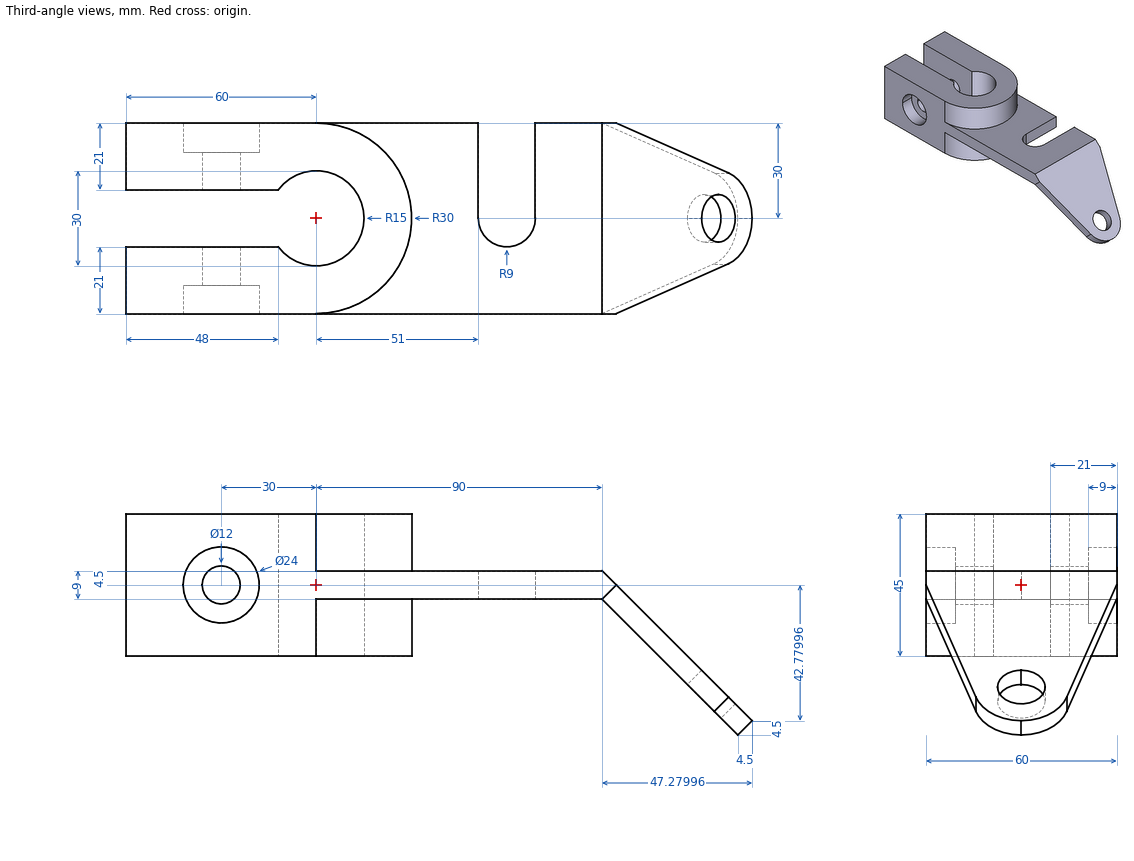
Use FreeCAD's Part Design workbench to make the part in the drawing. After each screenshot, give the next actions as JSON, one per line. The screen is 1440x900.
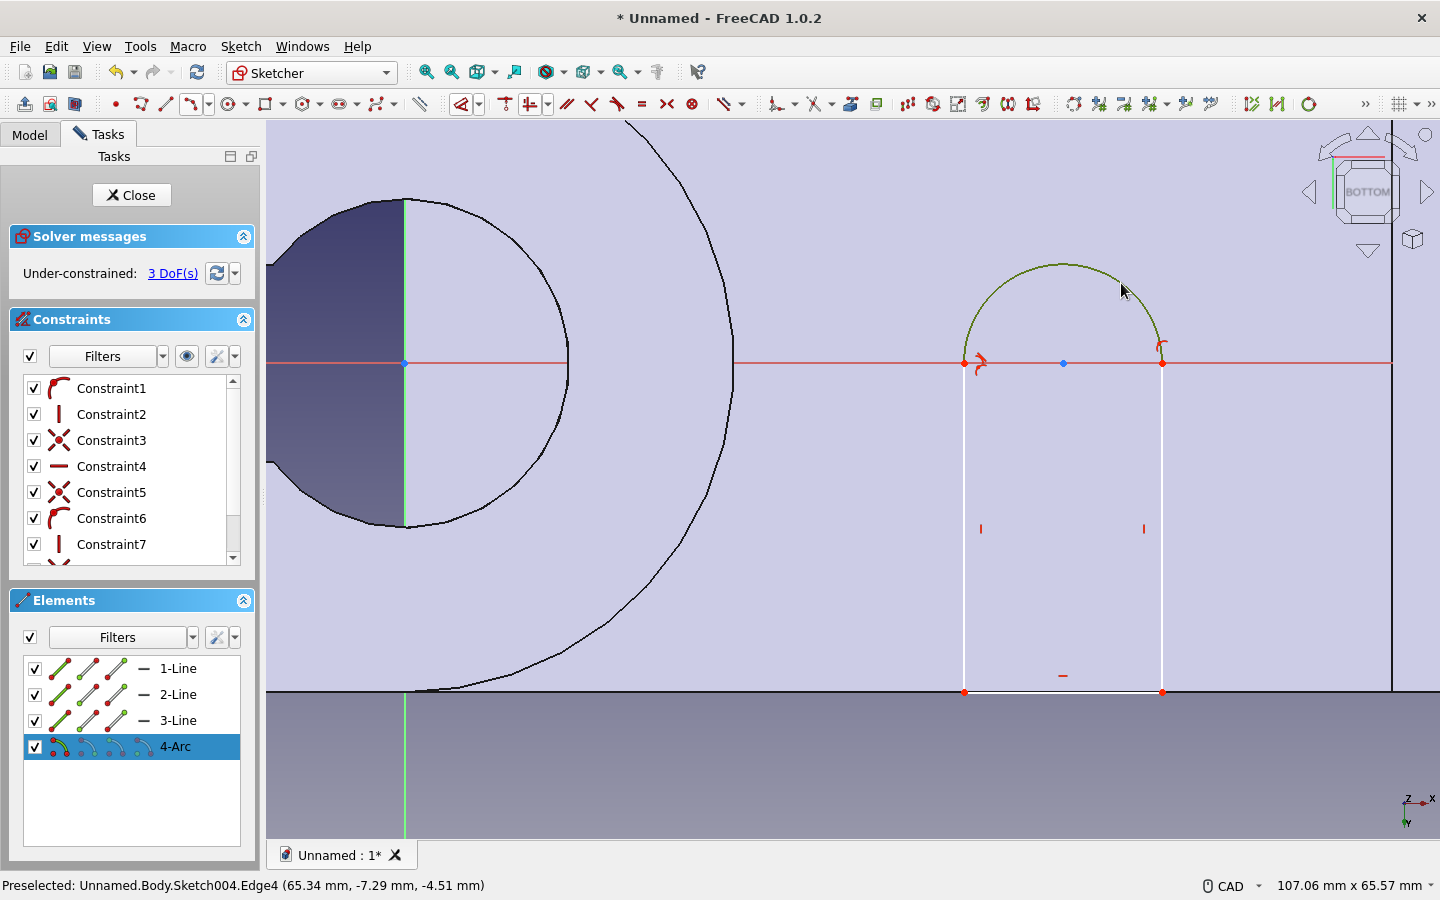
{"action": "left_click", "coordinate": [478, 104]}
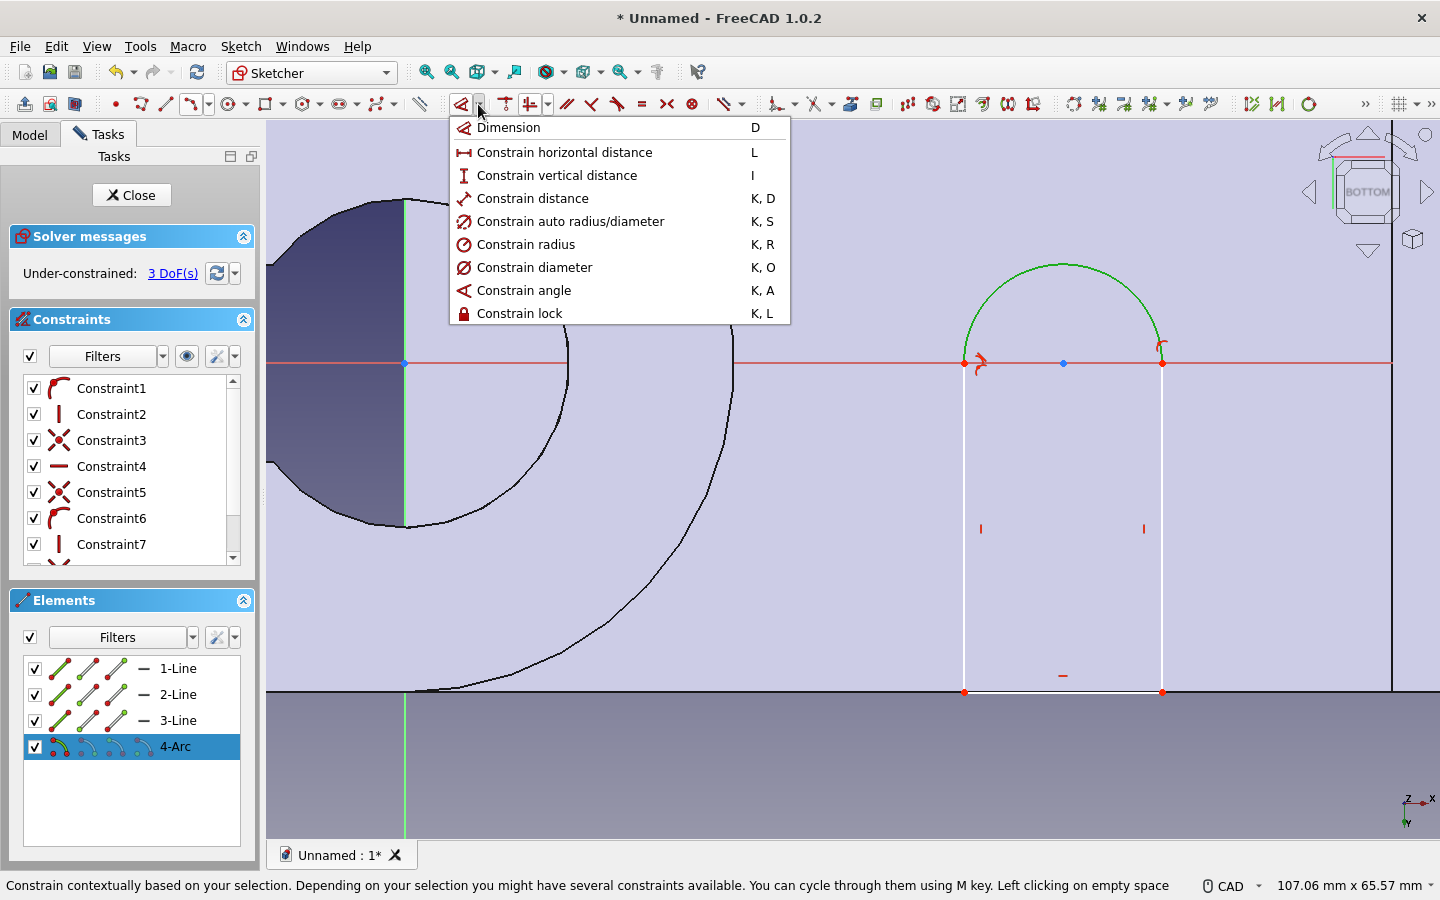
{"action": "left_click", "coordinate": [620, 244]}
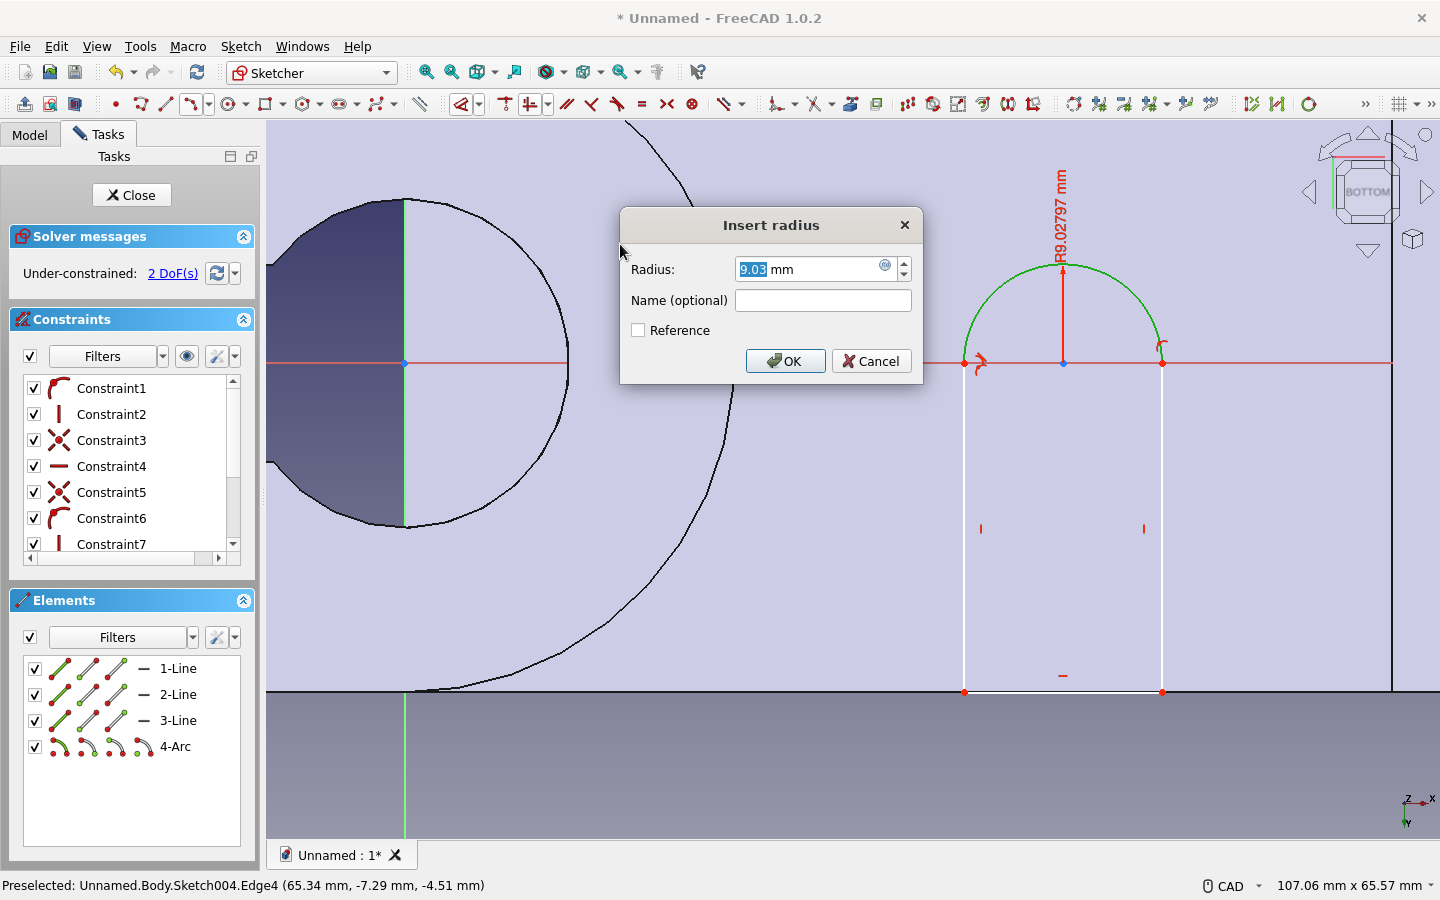
{"action": "type", "text": "9"}
{"action": "key", "text": "Return"}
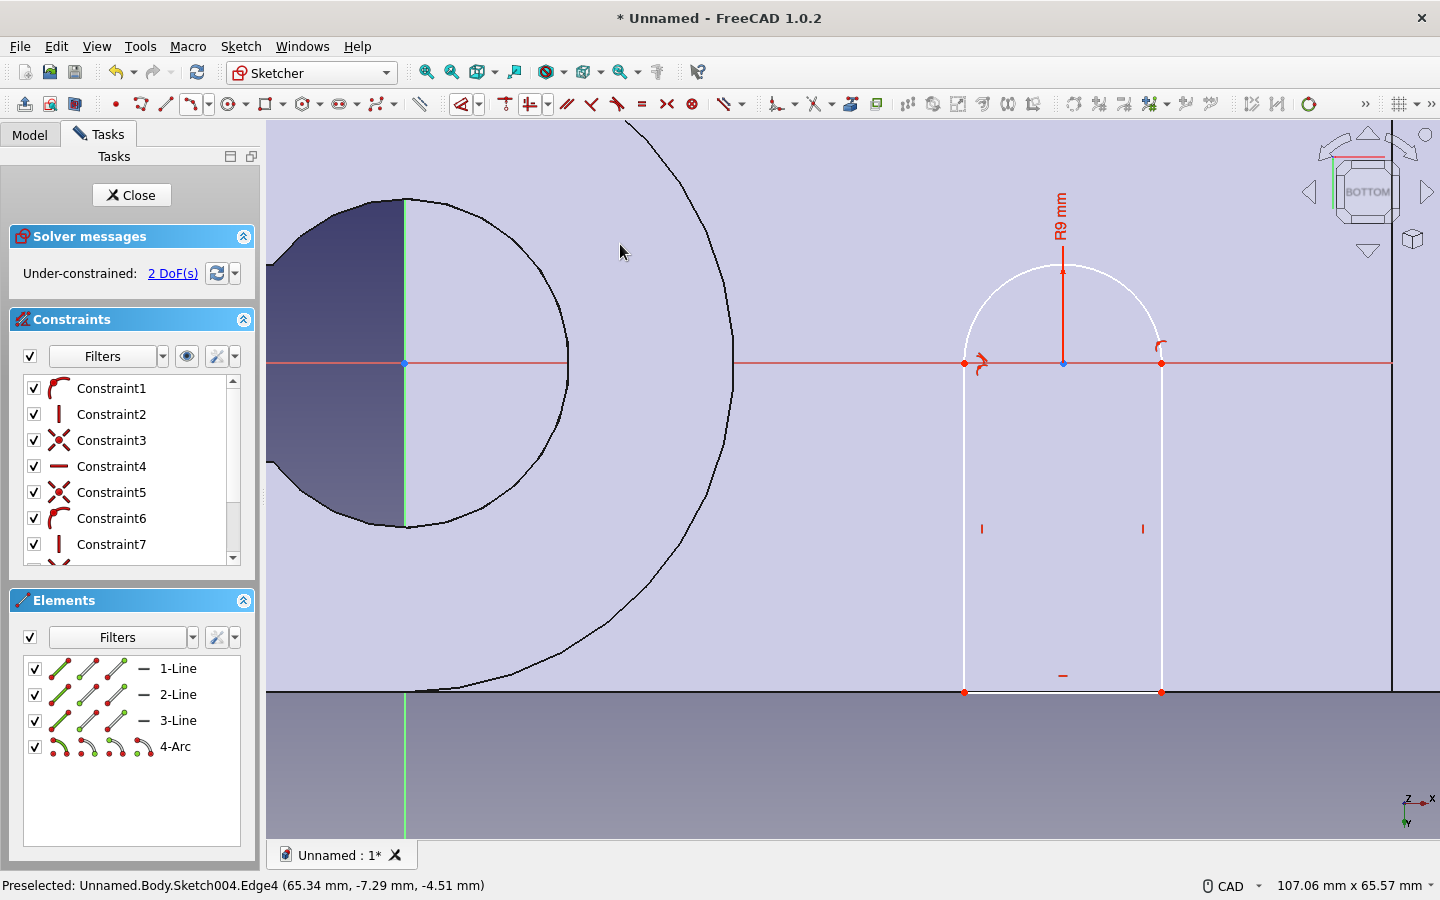
{"action": "left_click", "coordinate": [964, 462]}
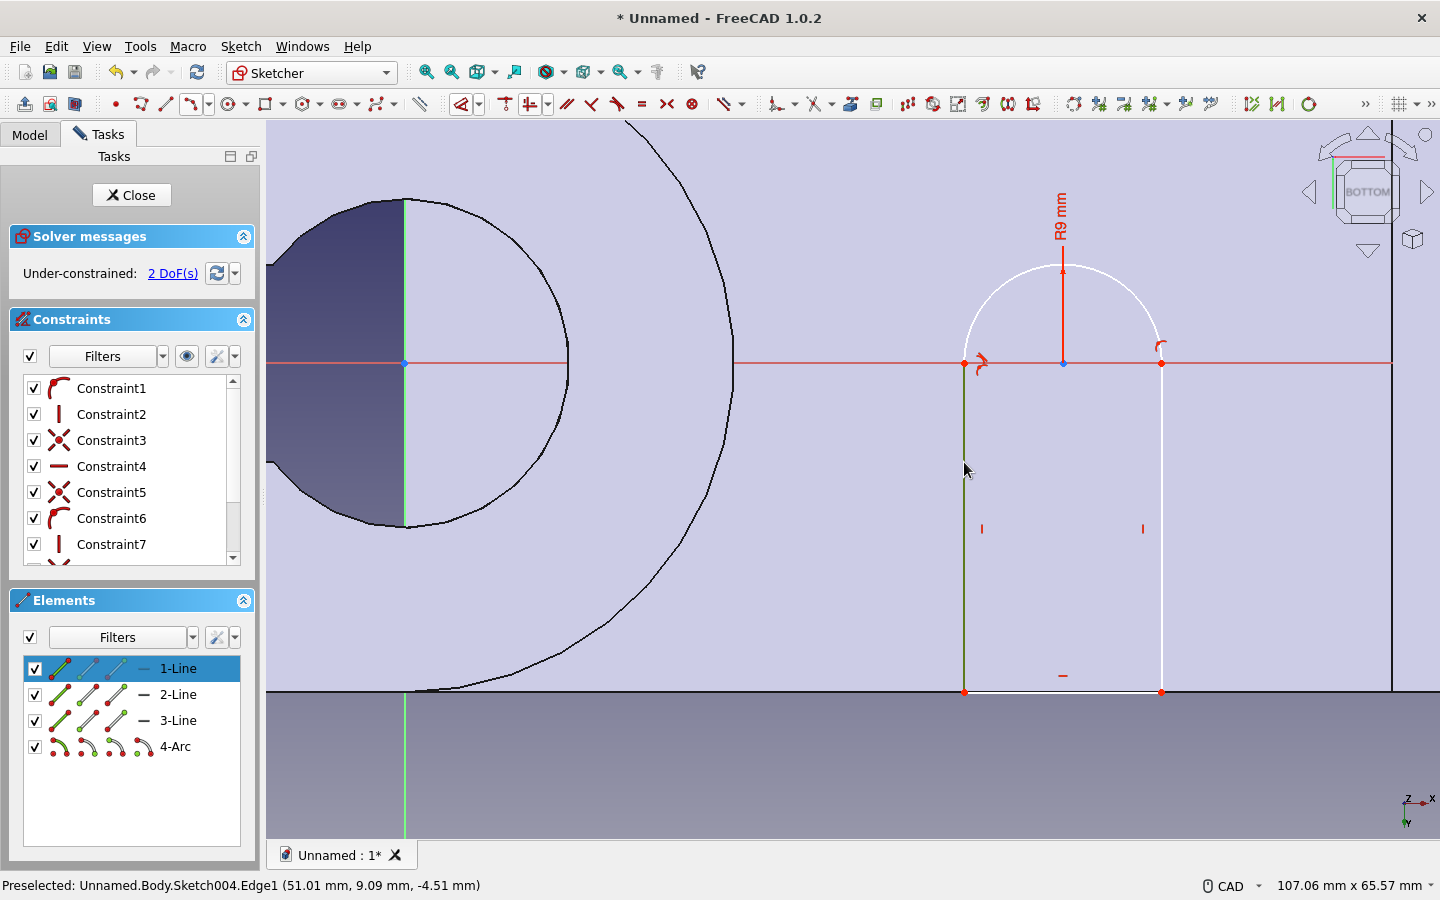
{"action": "key", "text": "i"}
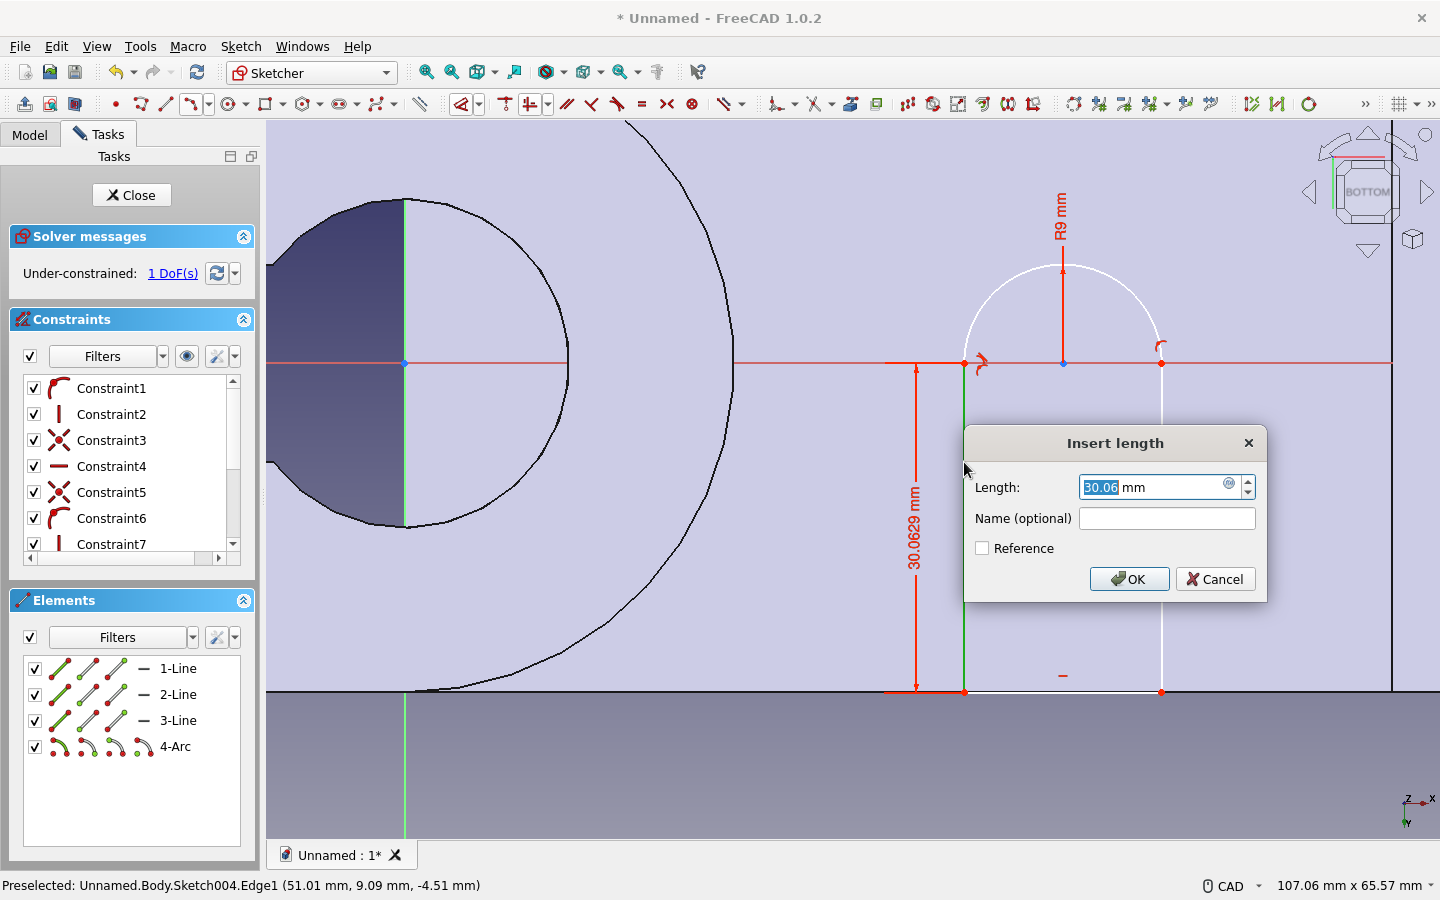
{"action": "type", "text": "30"}
{"action": "key", "text": "Return"}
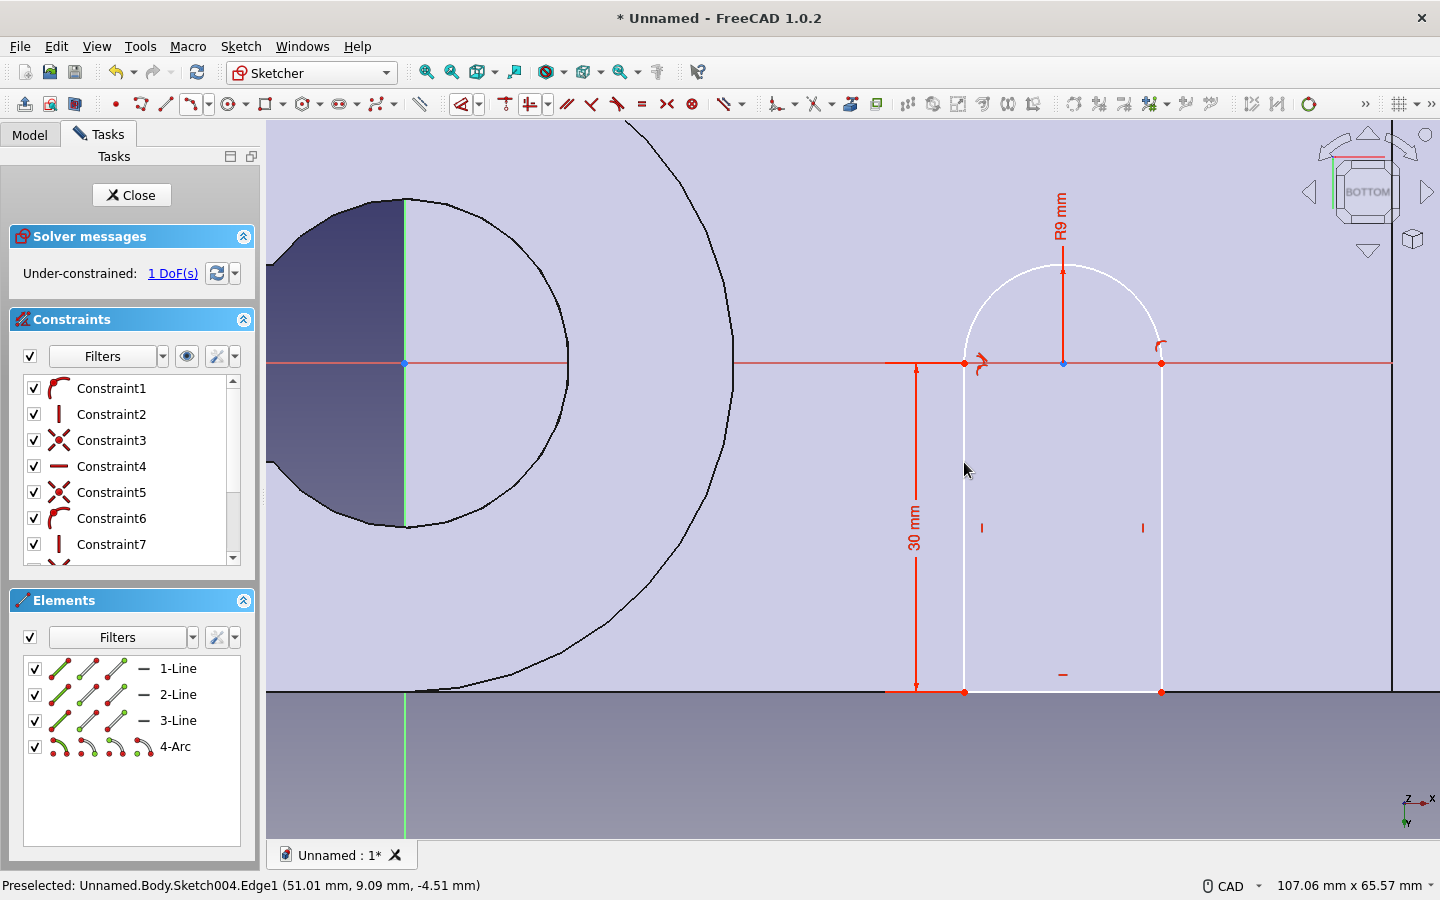
{"action": "left_click", "coordinate": [964, 363]}